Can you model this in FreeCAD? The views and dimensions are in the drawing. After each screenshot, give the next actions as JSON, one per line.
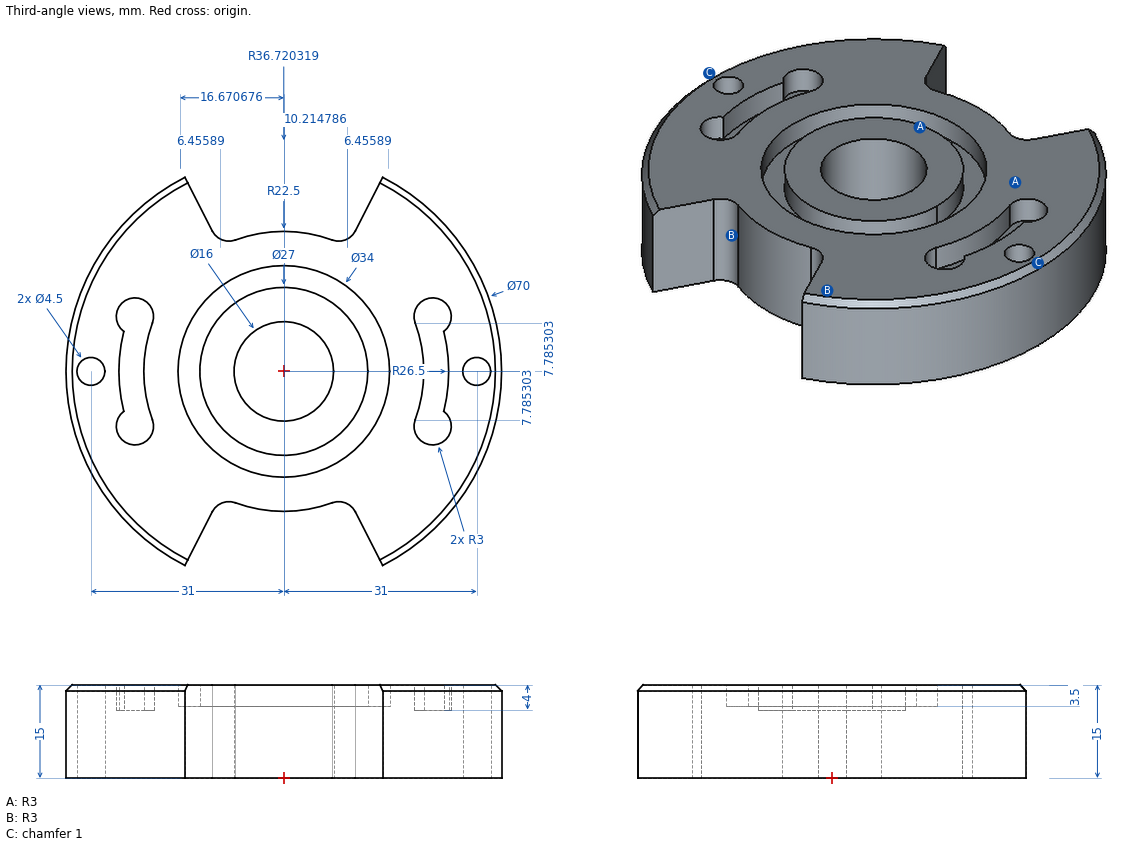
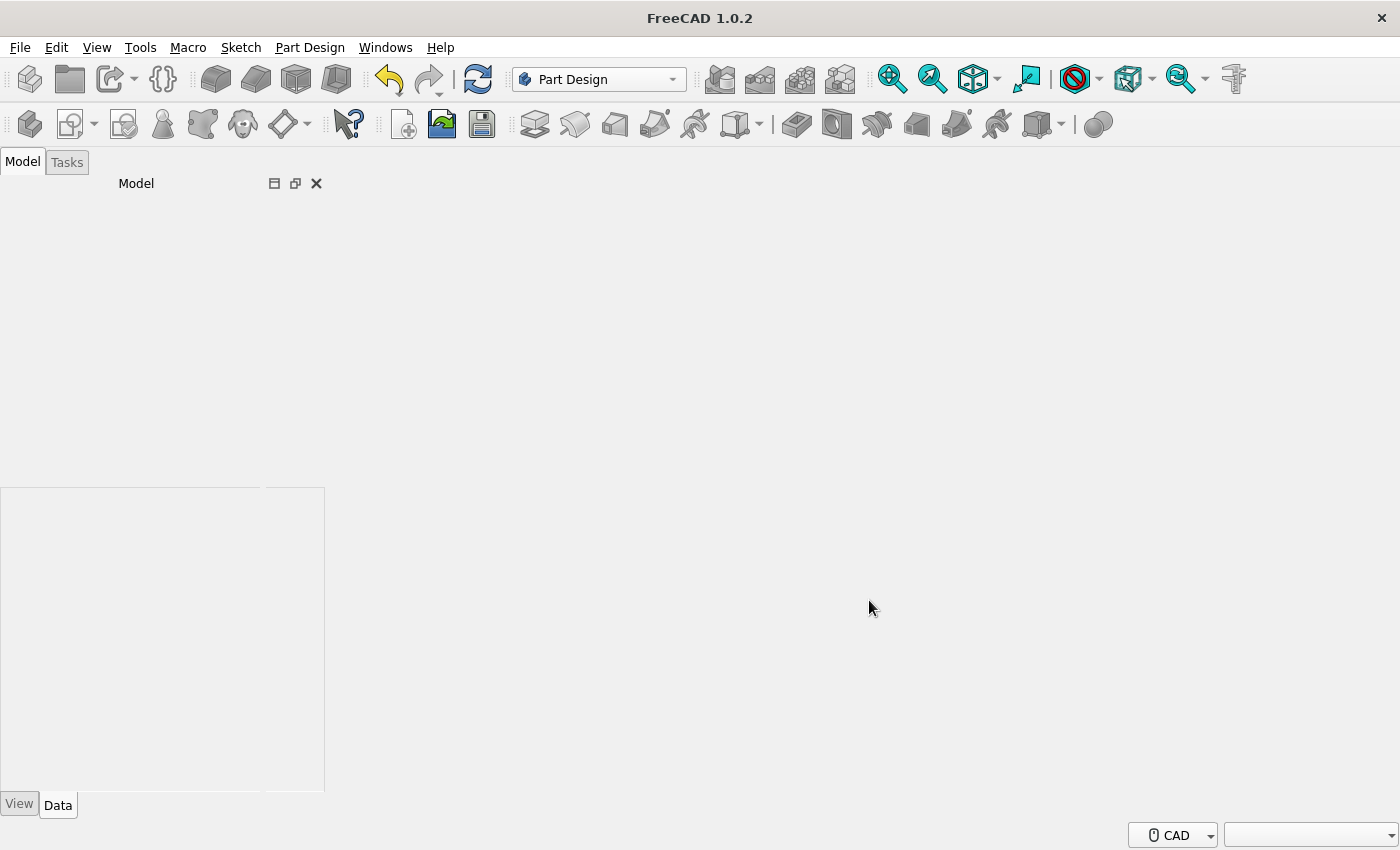
{"action": "left_click", "coordinate": [402, 124]}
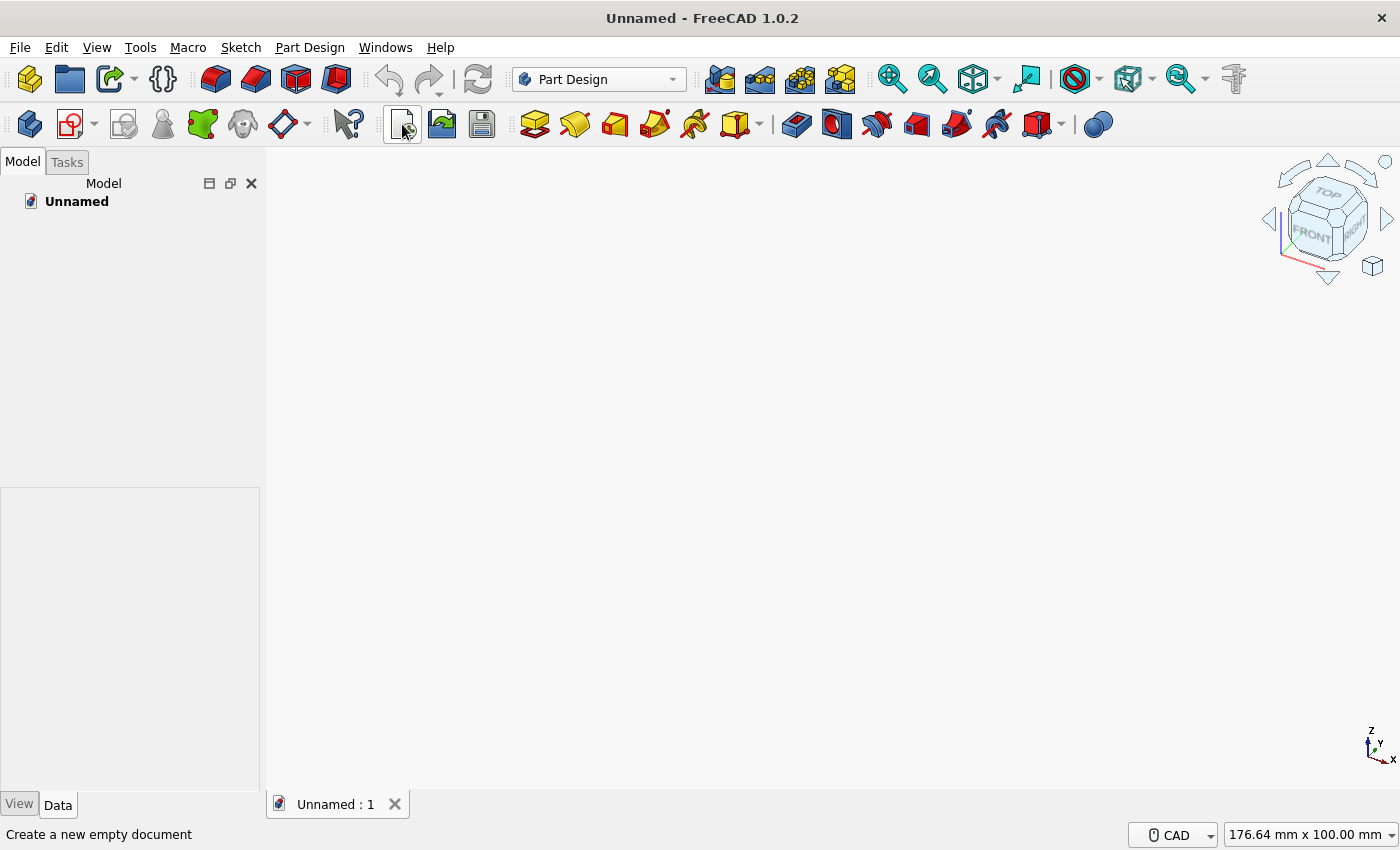
{"action": "left_click", "coordinate": [70, 124]}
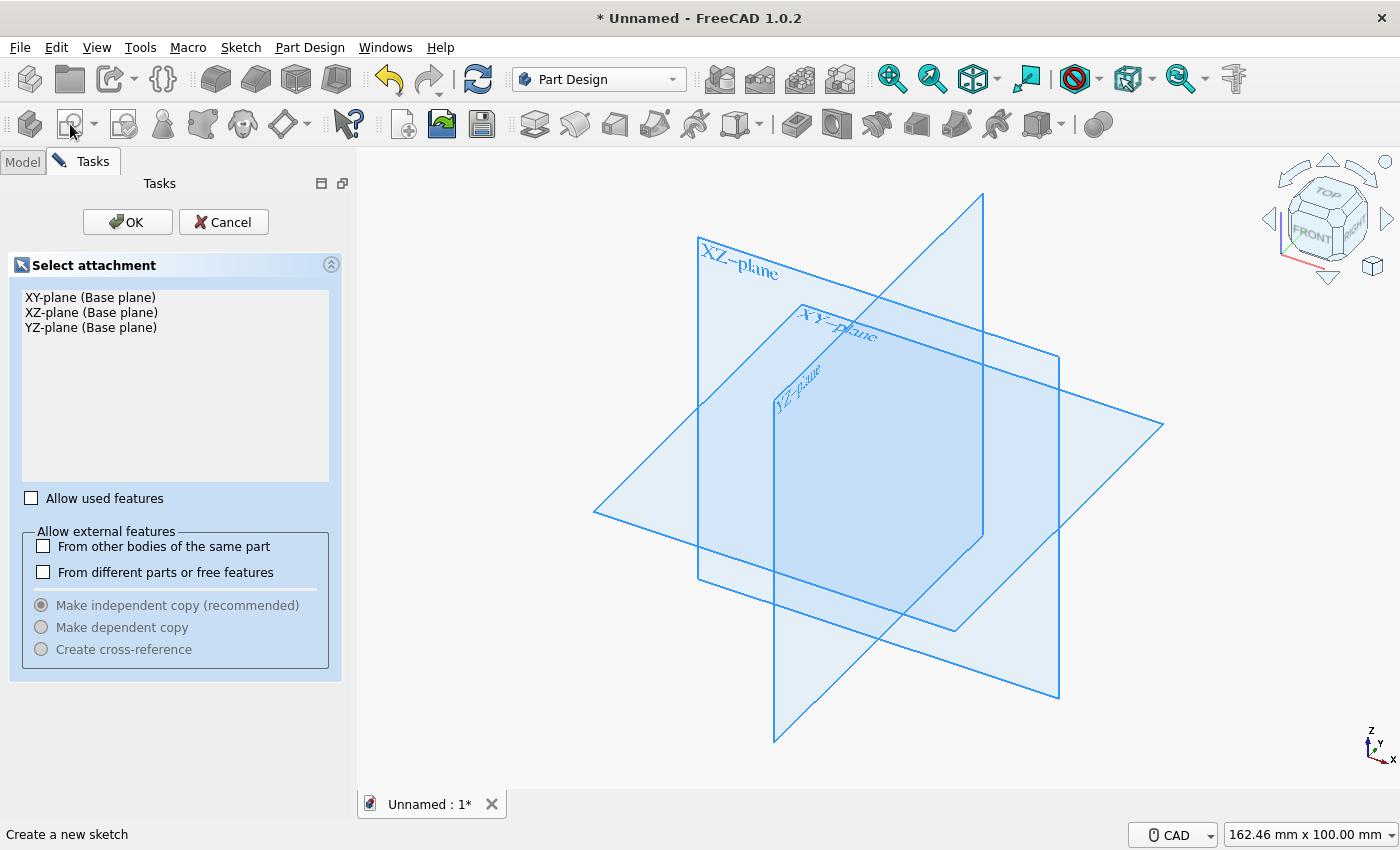
{"action": "left_click", "coordinate": [82, 298]}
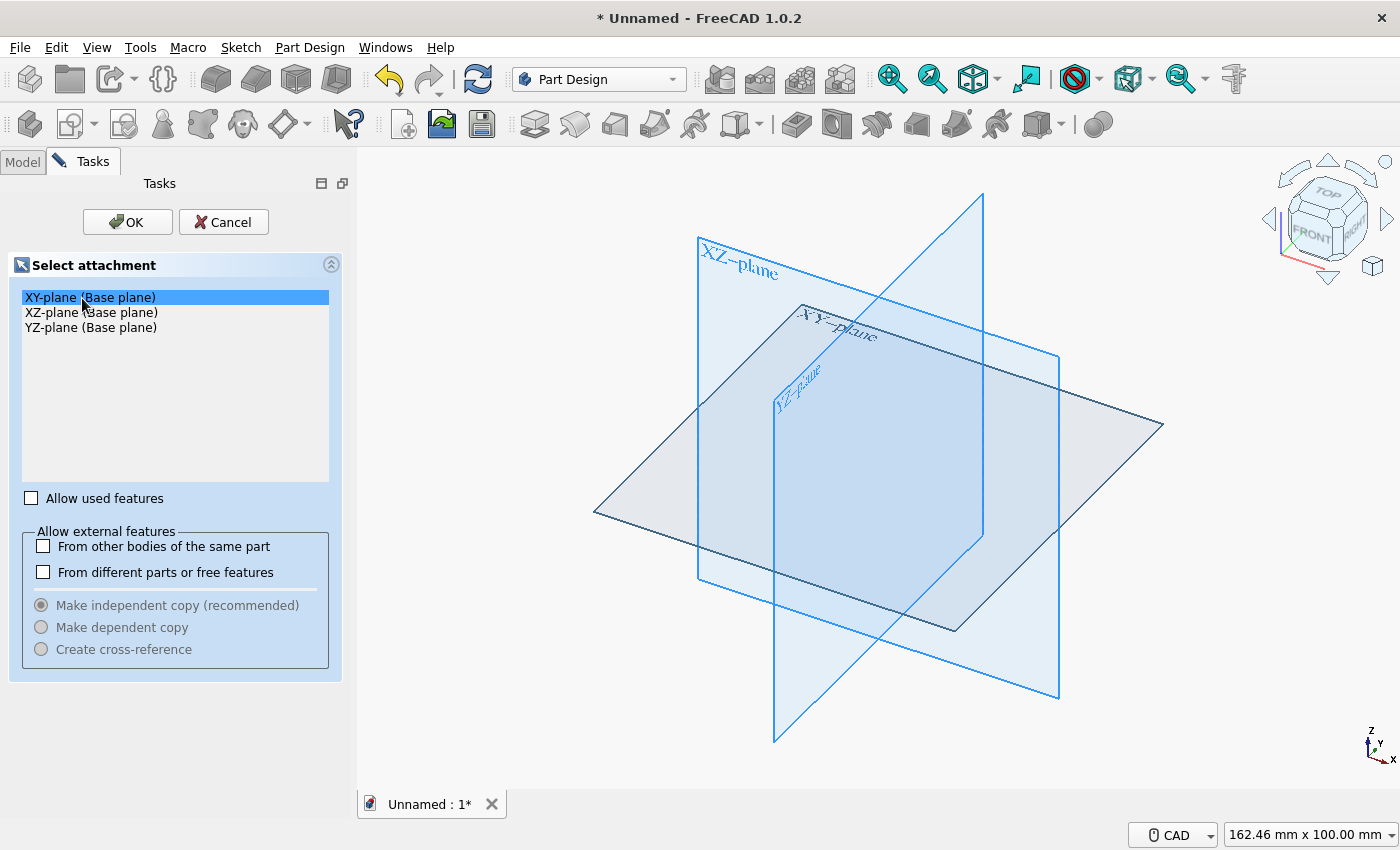
{"action": "left_click", "coordinate": [128, 222]}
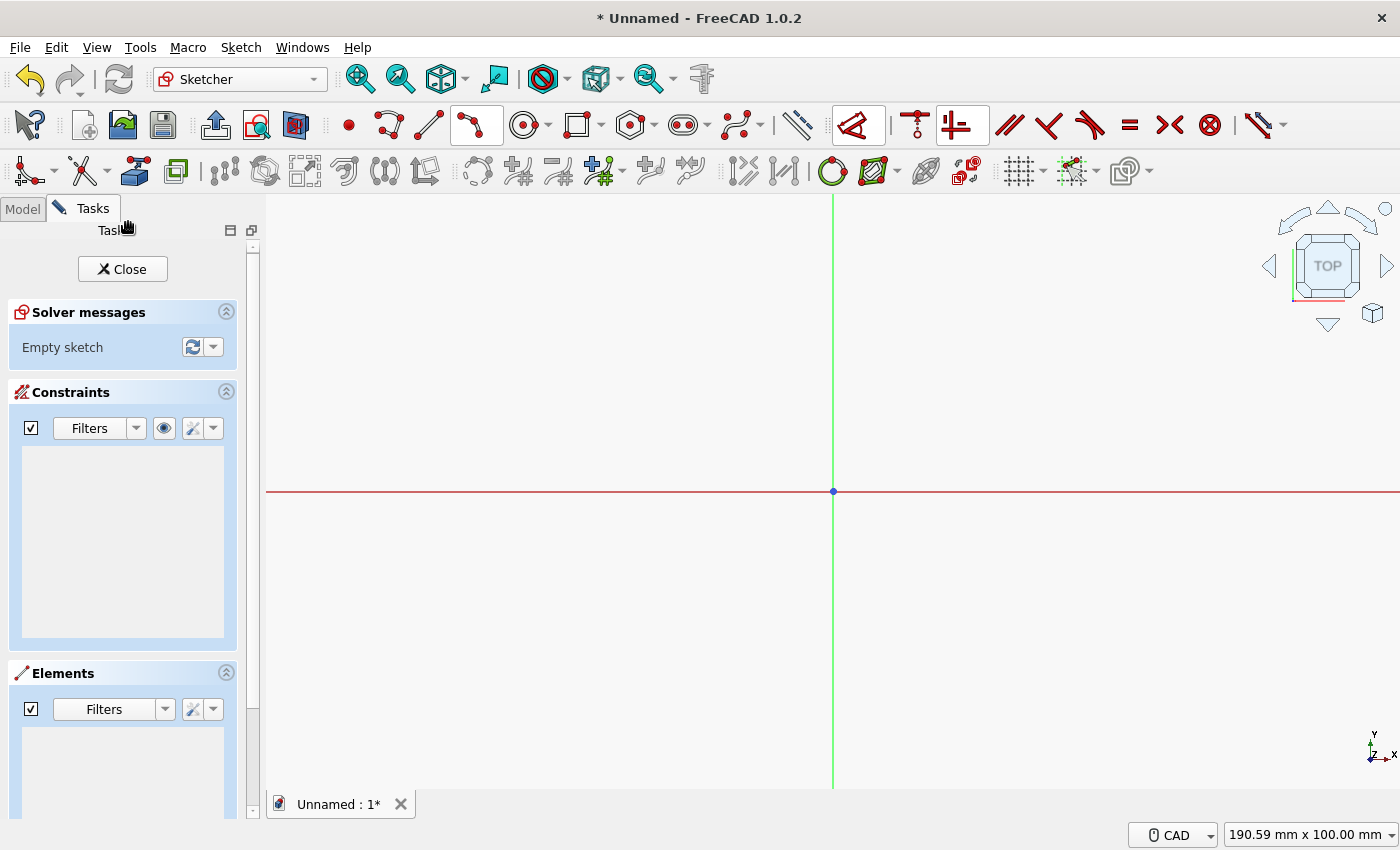
{"action": "left_click", "coordinate": [524, 126]}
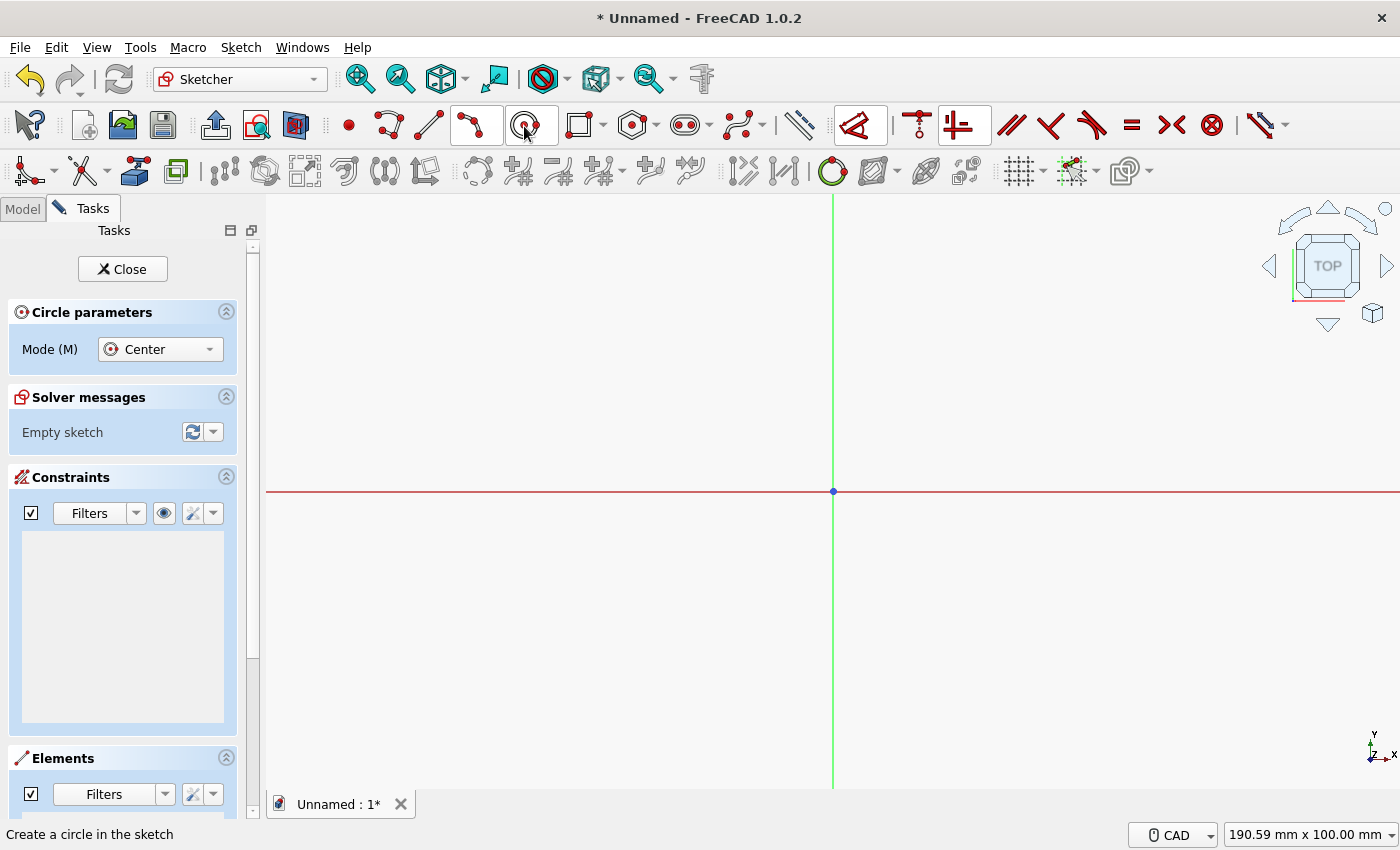
{"action": "left_click", "coordinate": [833, 492]}
{"action": "mouse_move", "coordinate": [980, 344]}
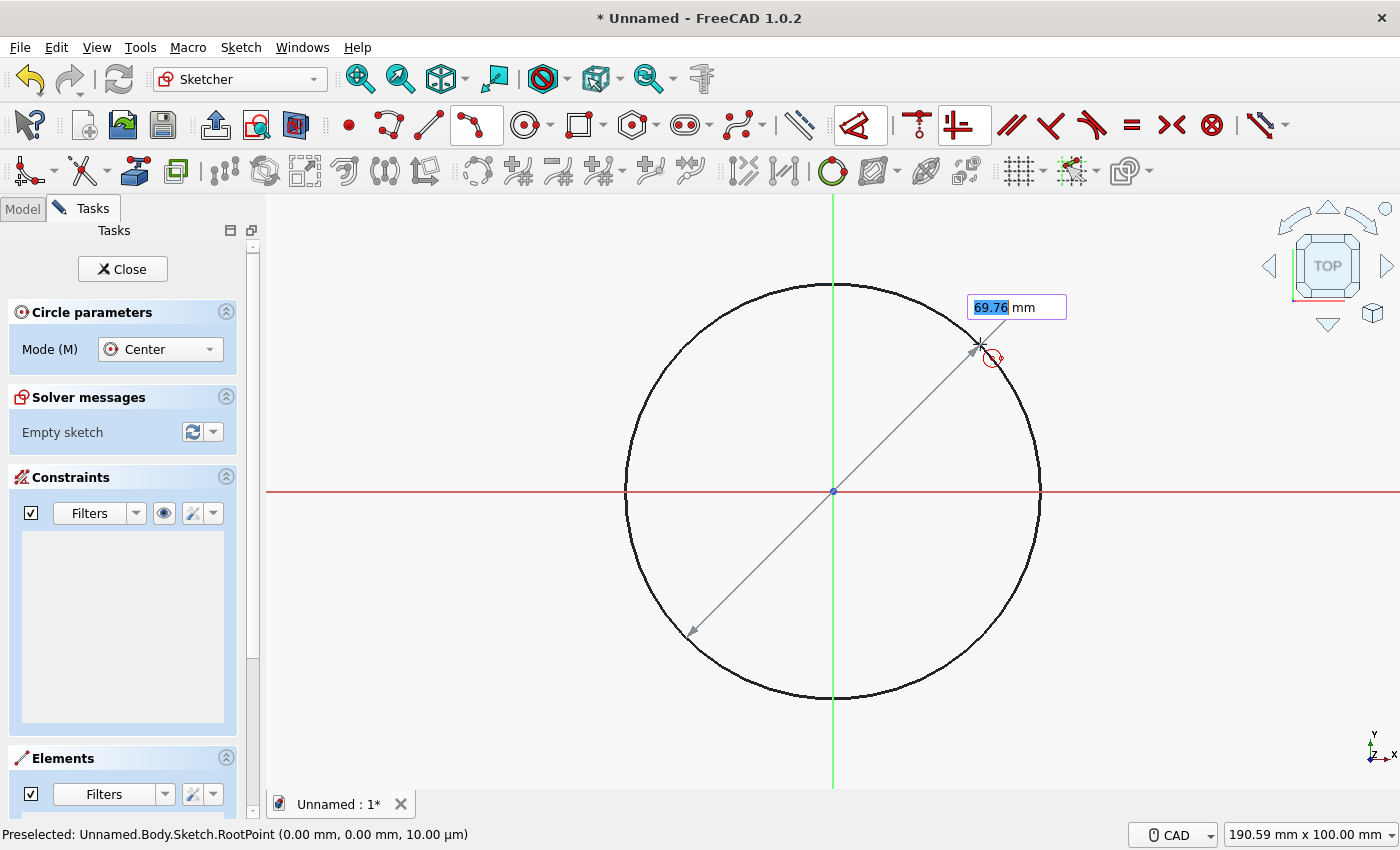
{"action": "type", "text": "70"}
{"action": "key", "text": "Return"}
{"action": "key", "text": "Escape"}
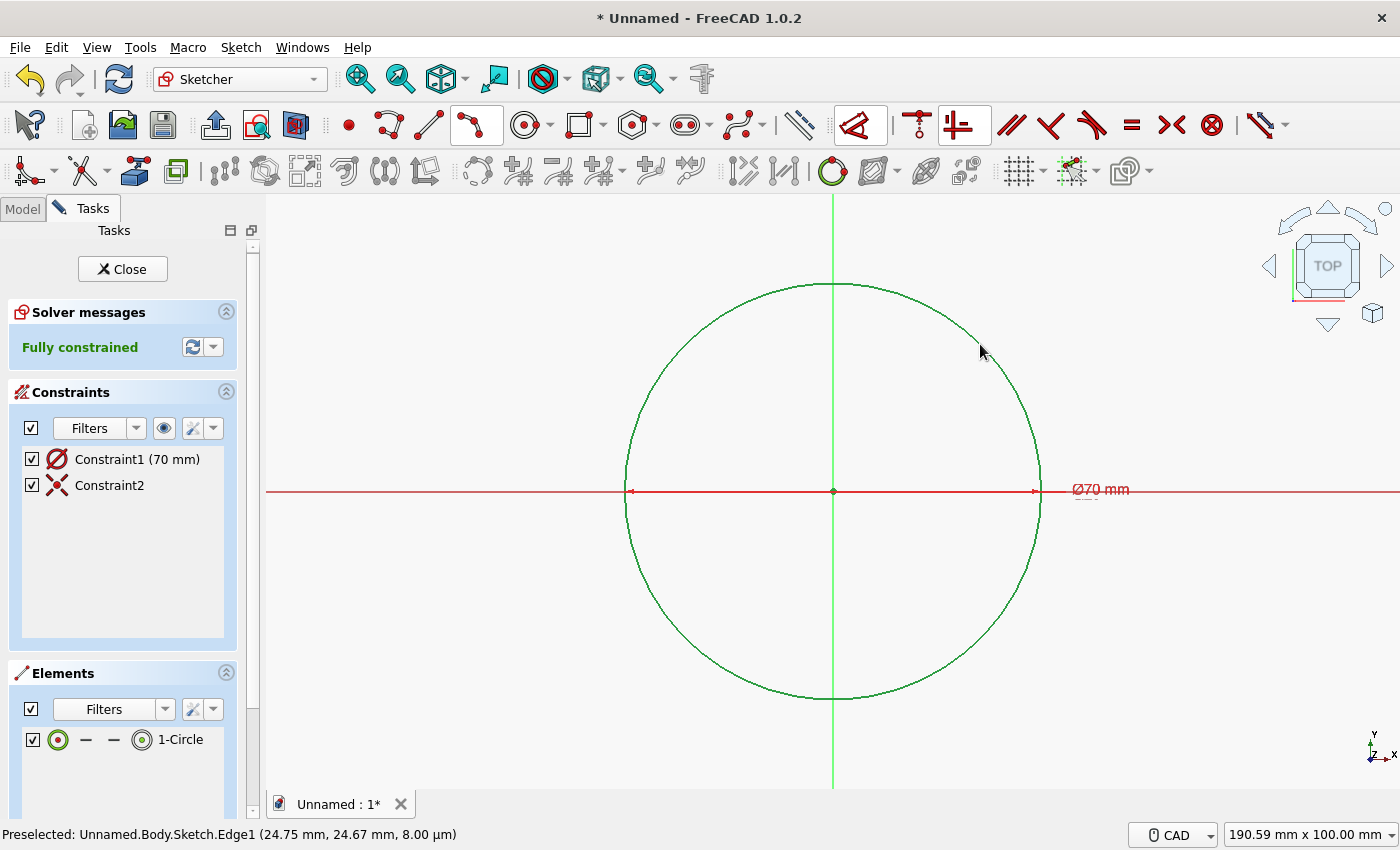
{"action": "left_click", "coordinate": [123, 269]}